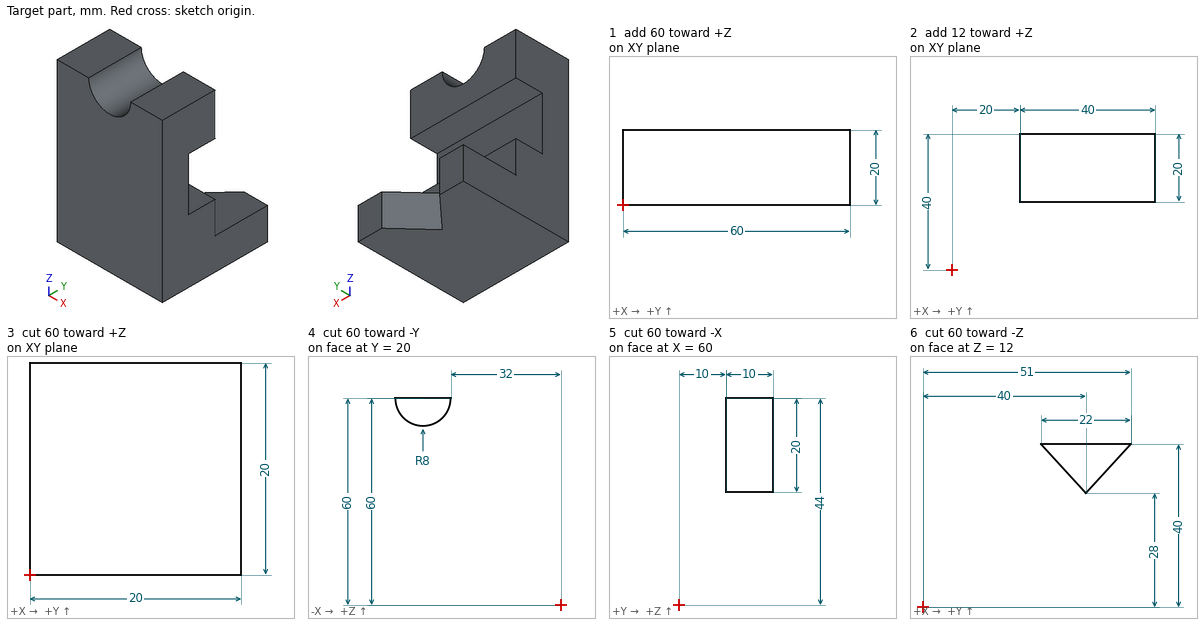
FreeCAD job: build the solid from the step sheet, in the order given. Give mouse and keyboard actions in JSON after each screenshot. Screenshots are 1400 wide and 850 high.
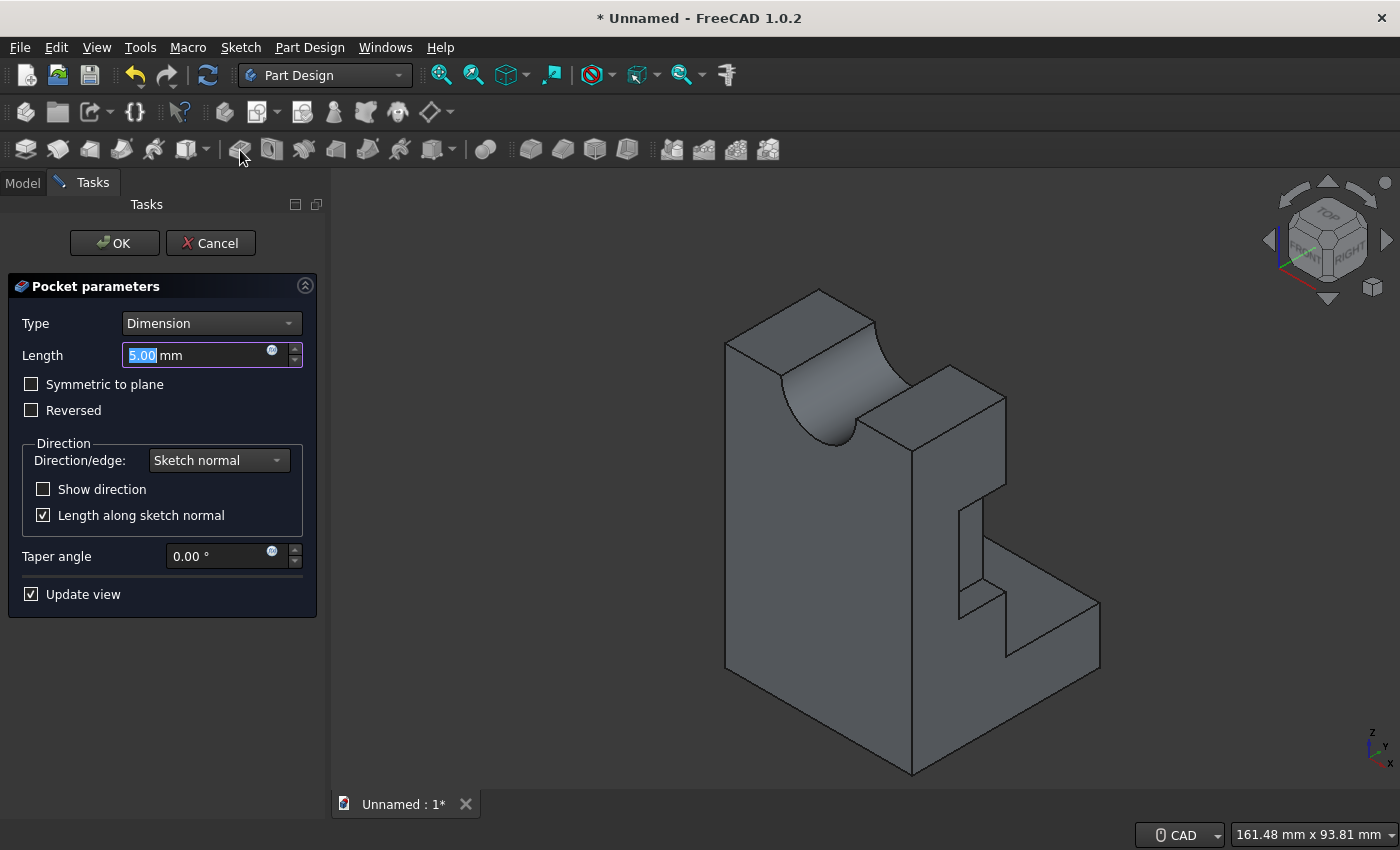
{"action": "type", "text": "60"}
{"action": "key", "text": "Tab"}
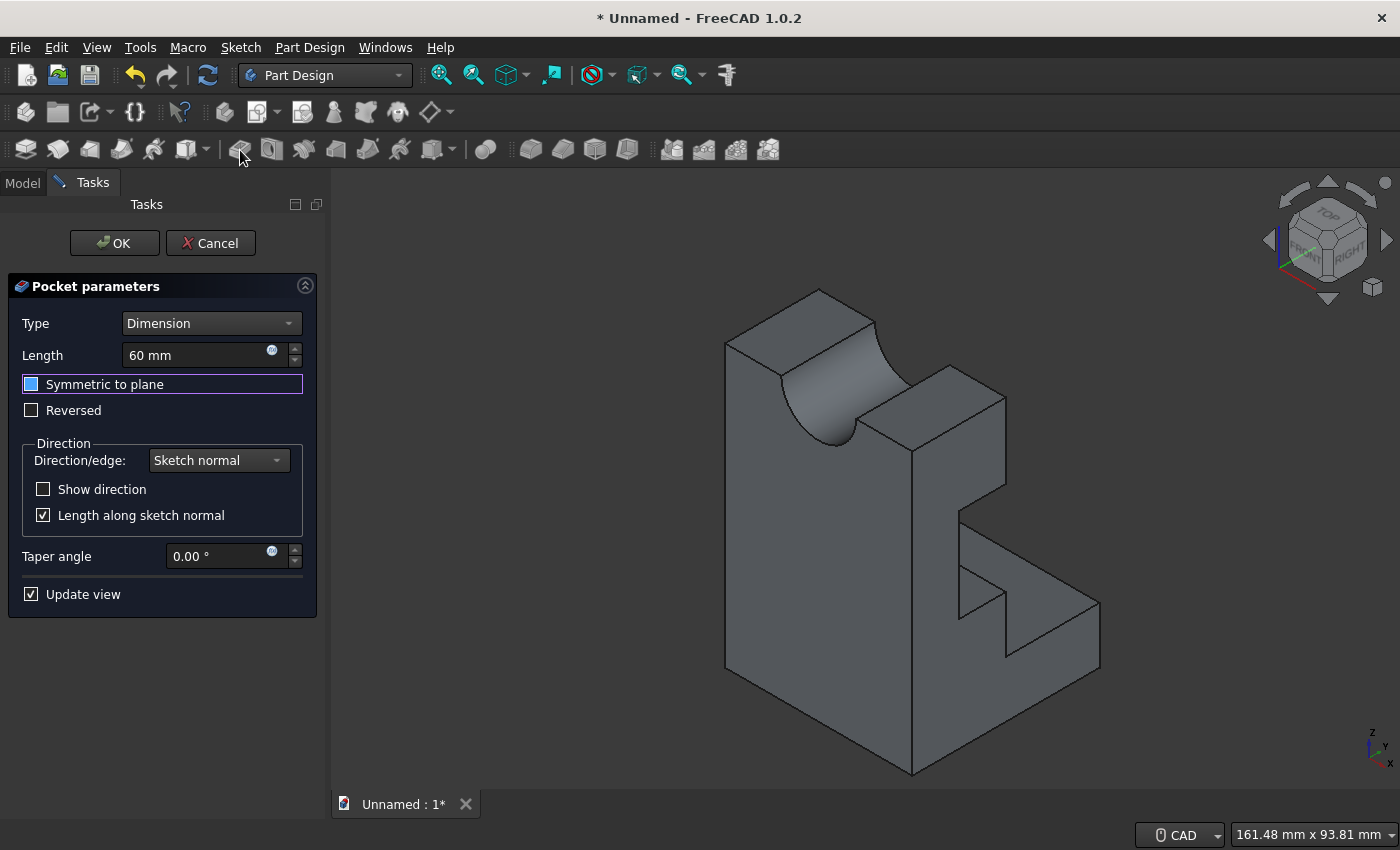
{"action": "left_click", "coordinate": [115, 243]}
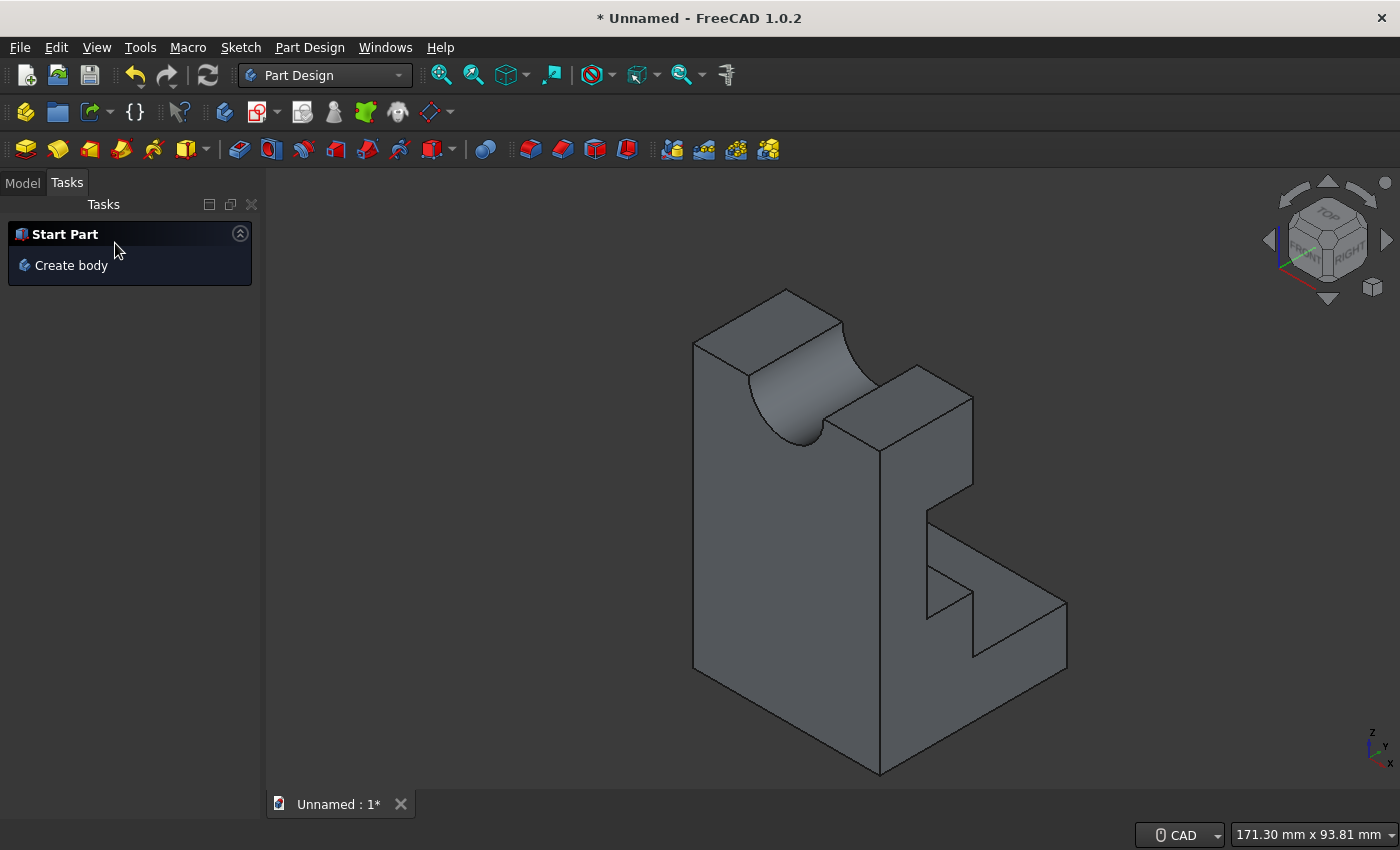
{"action": "key", "text": "2"}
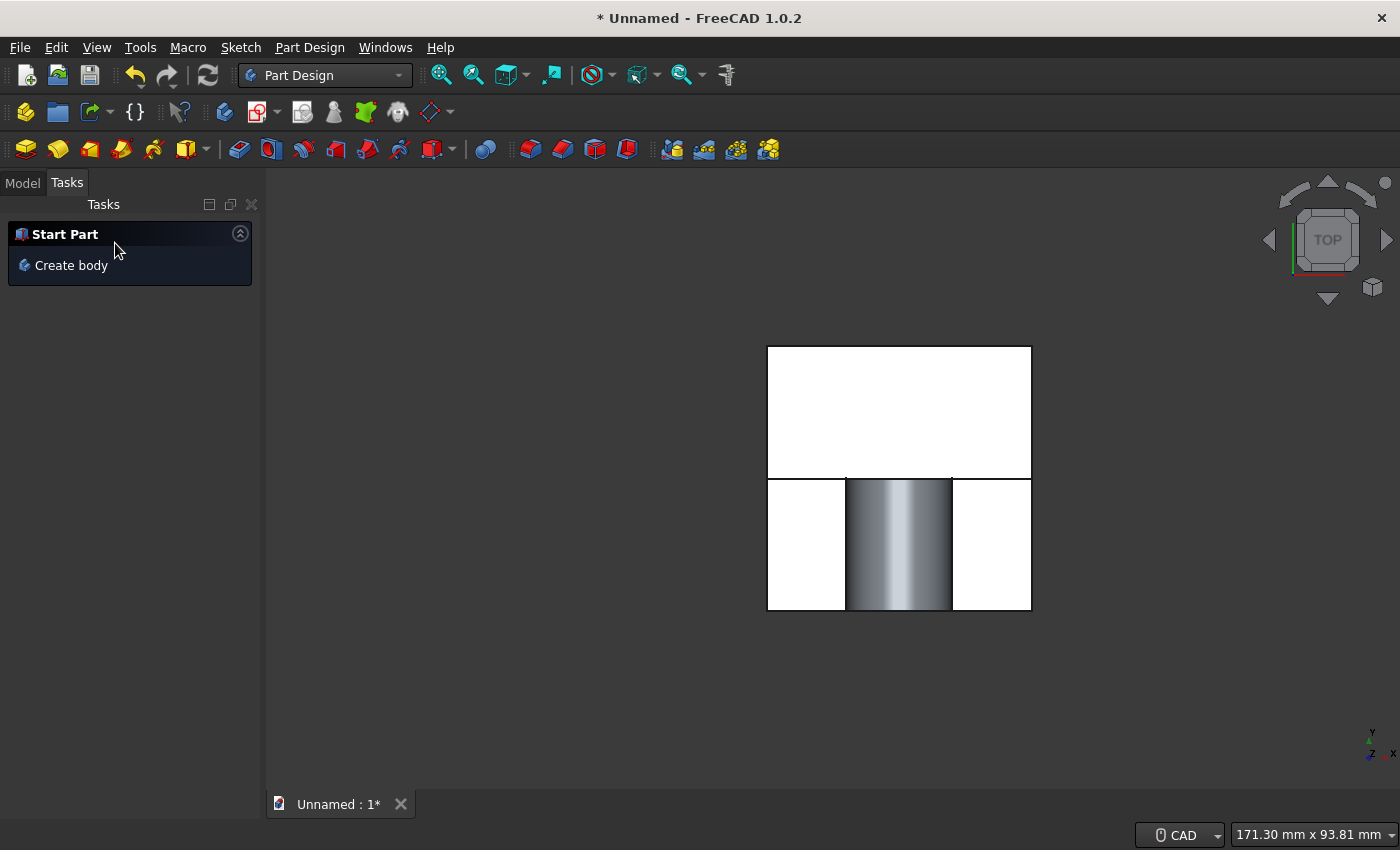
{"action": "left_click", "coordinate": [442, 76]}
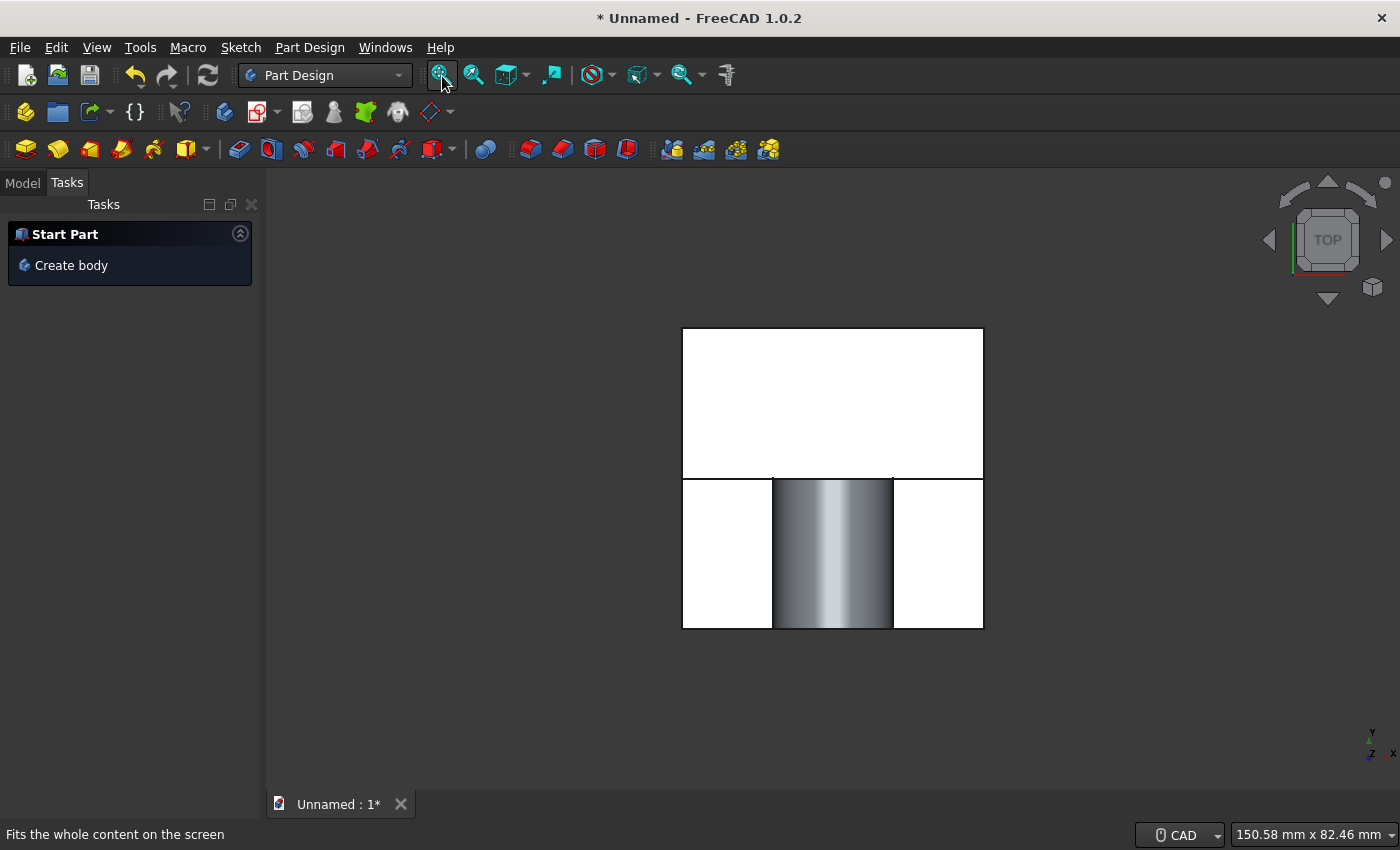
{"action": "left_click", "coordinate": [876, 402]}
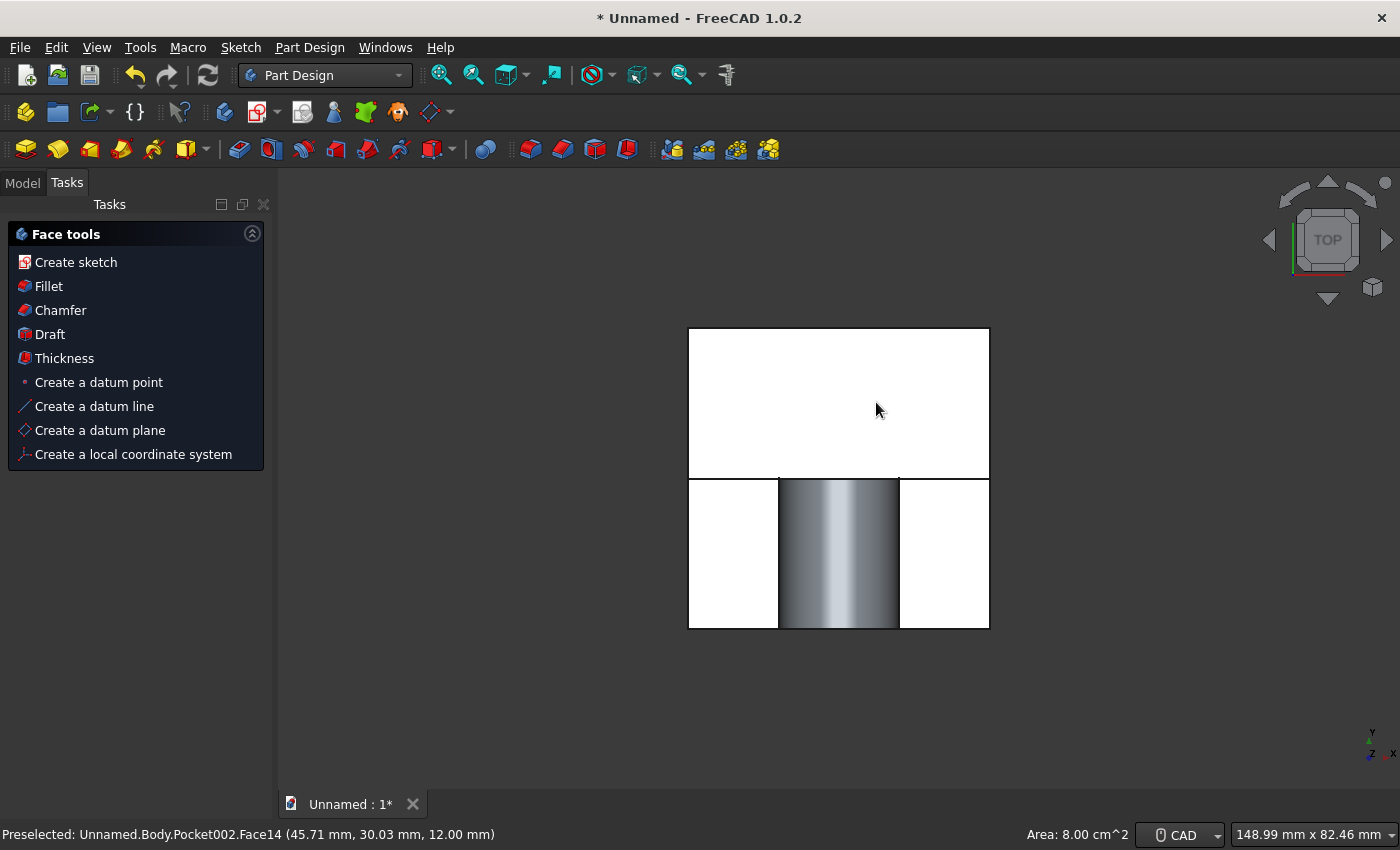
{"action": "left_click", "coordinate": [258, 112]}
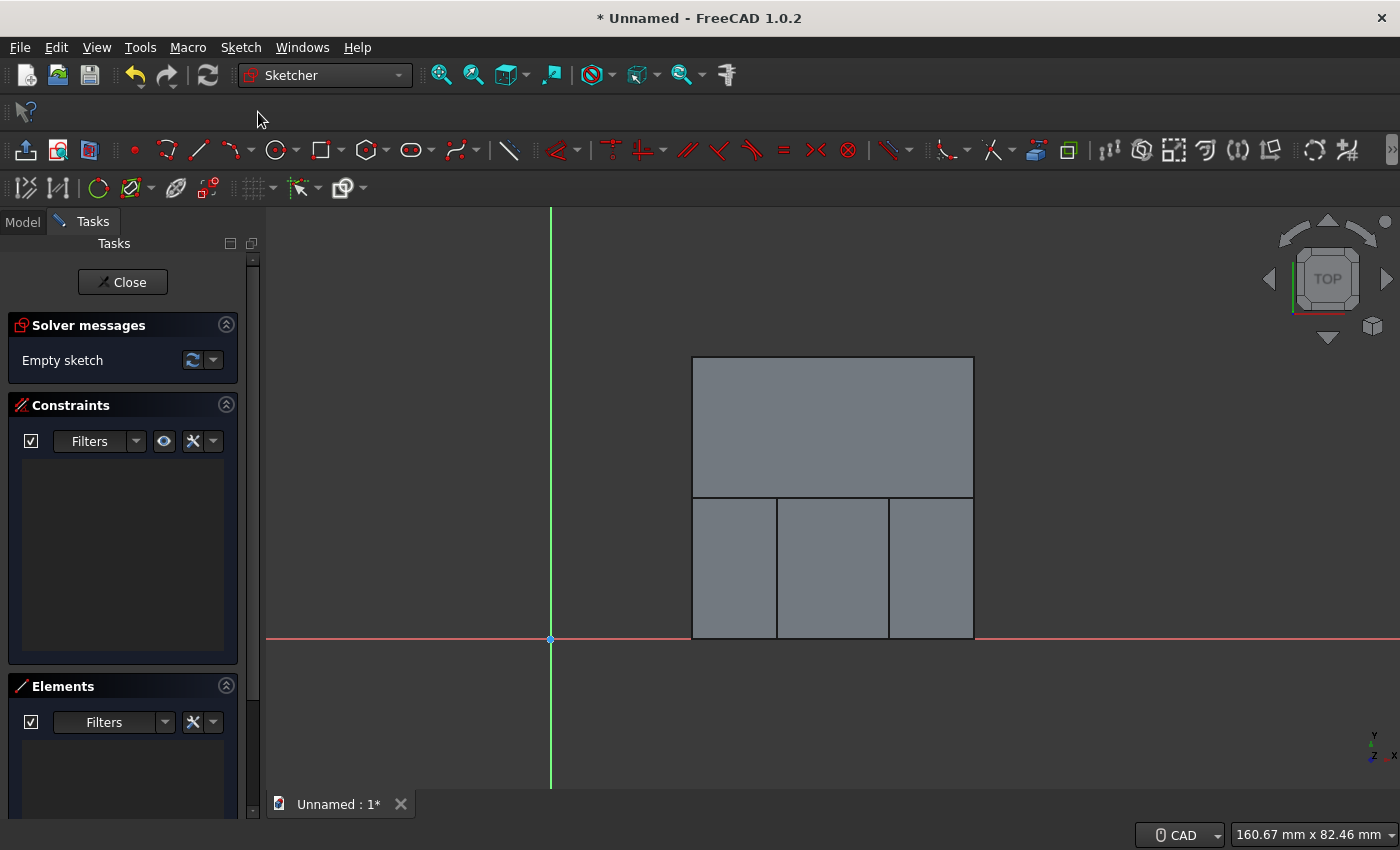
{"action": "left_click", "coordinate": [90, 150]}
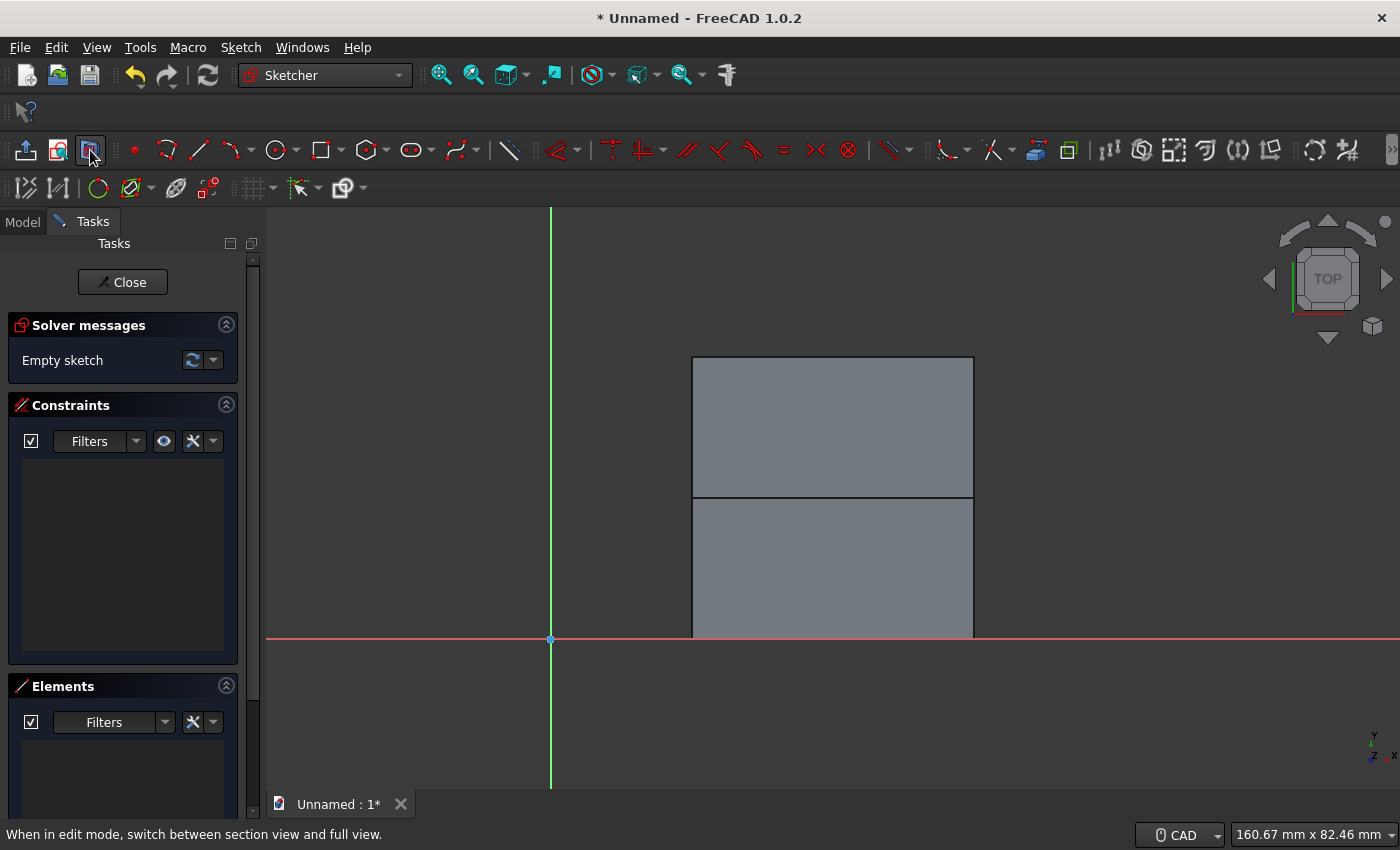
{"action": "left_click", "coordinate": [168, 150]}